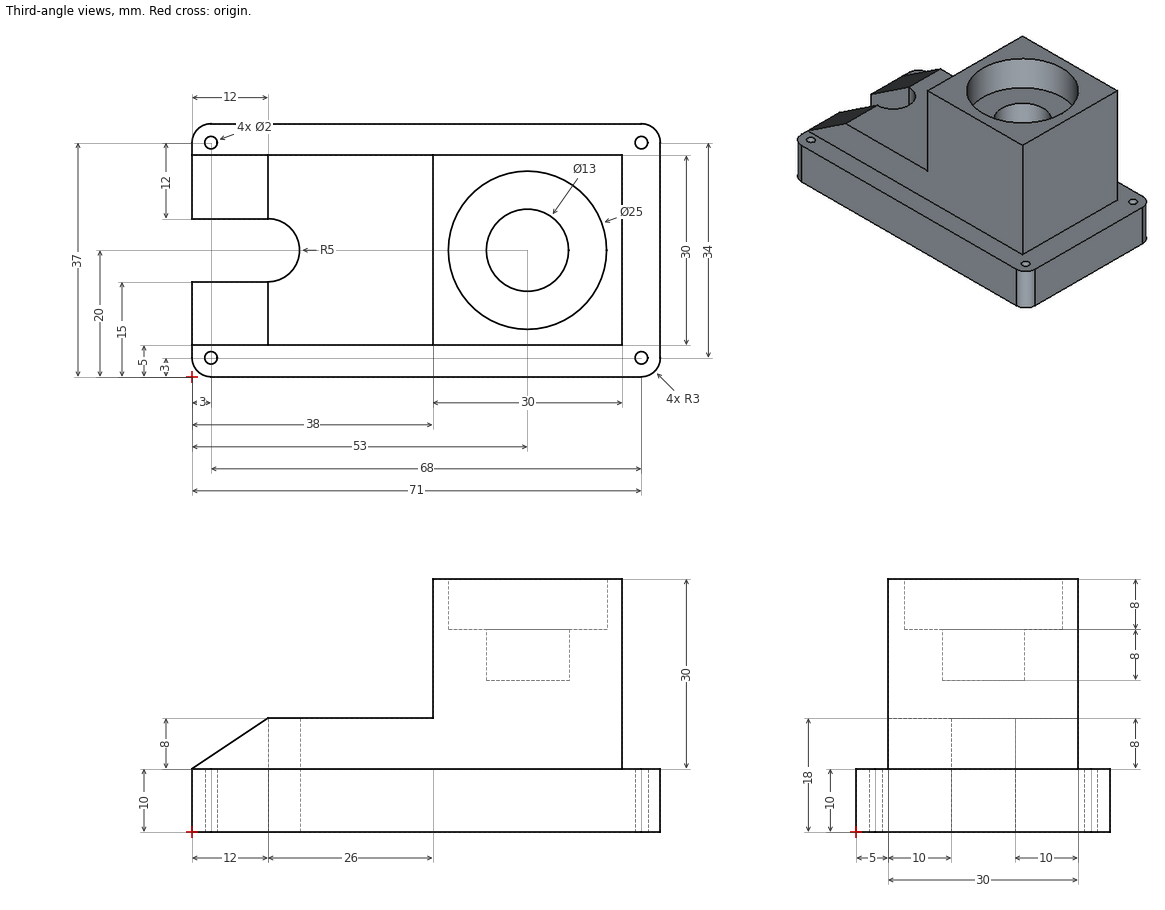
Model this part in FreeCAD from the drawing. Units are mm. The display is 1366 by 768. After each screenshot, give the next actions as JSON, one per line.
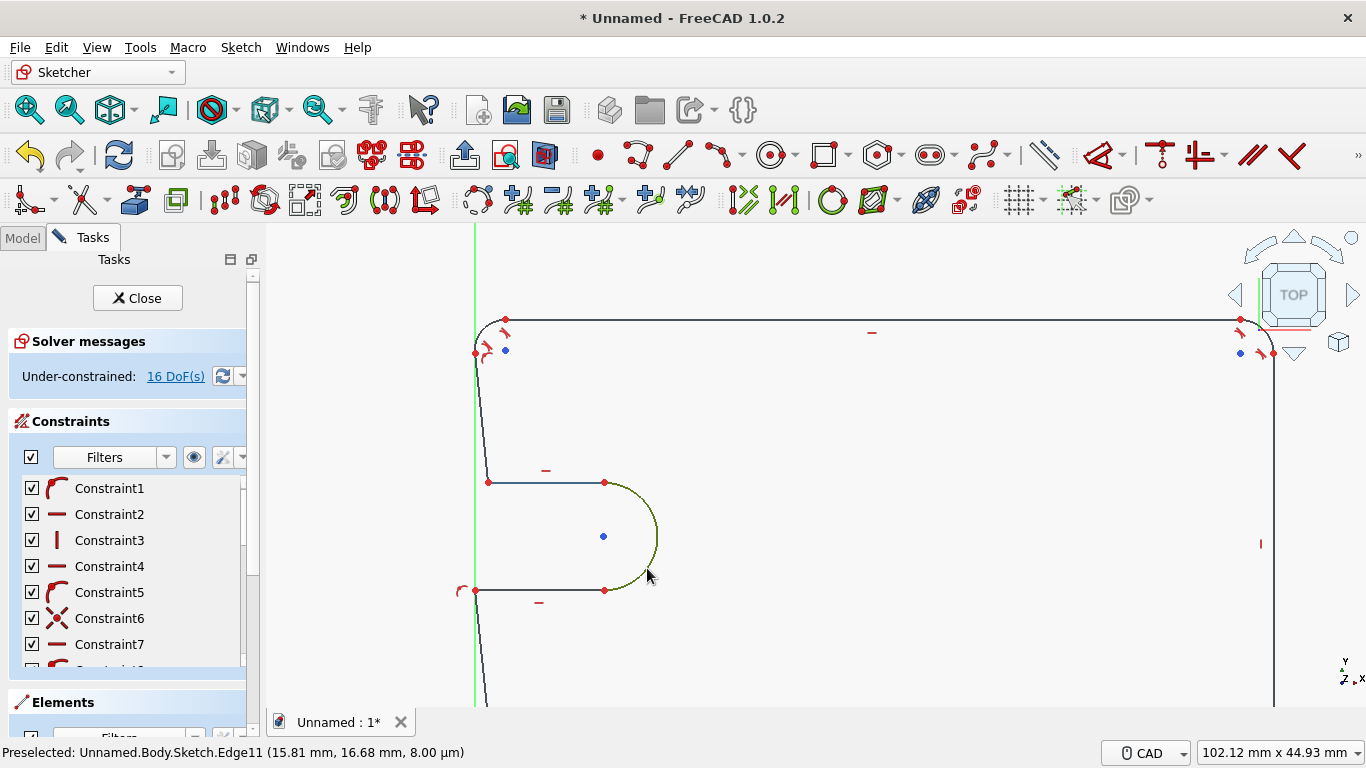
{"action": "key", "text": "t"}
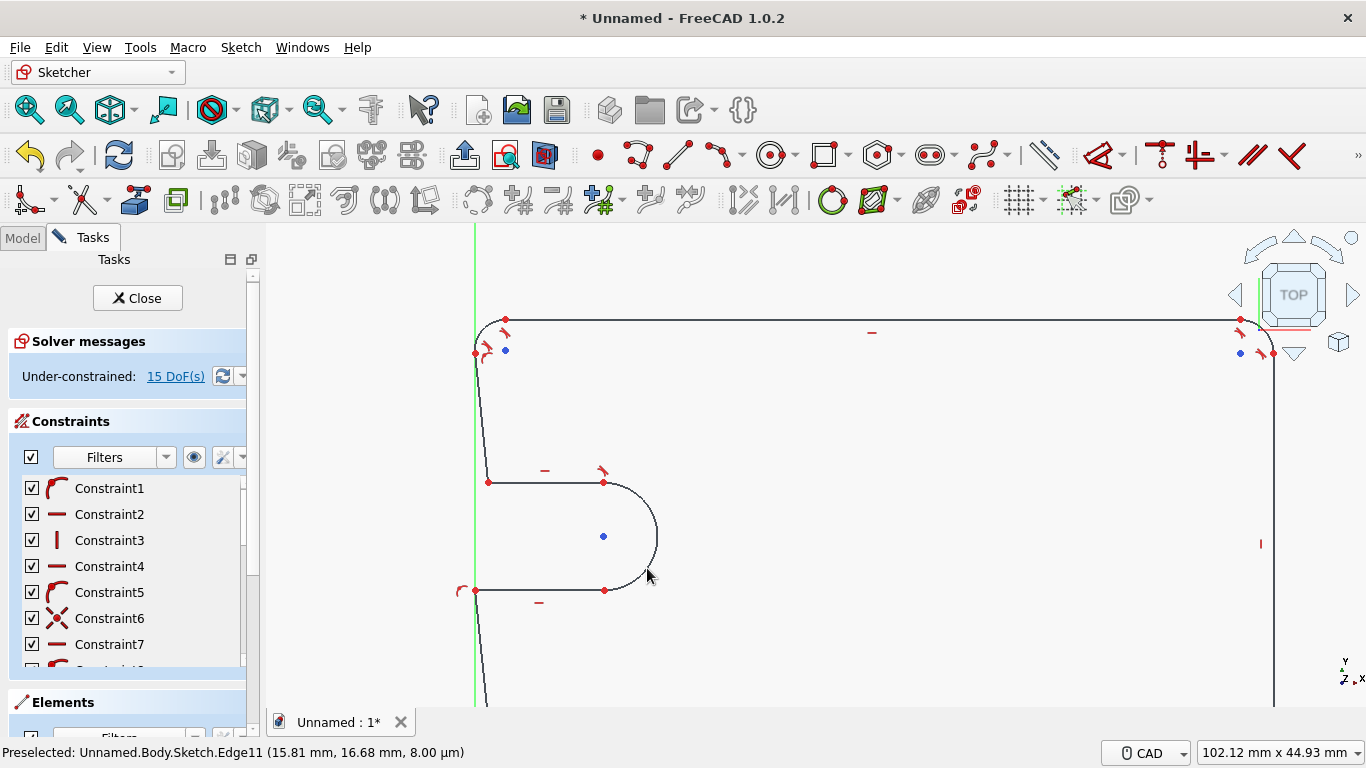
{"action": "left_click", "coordinate": [566, 590]}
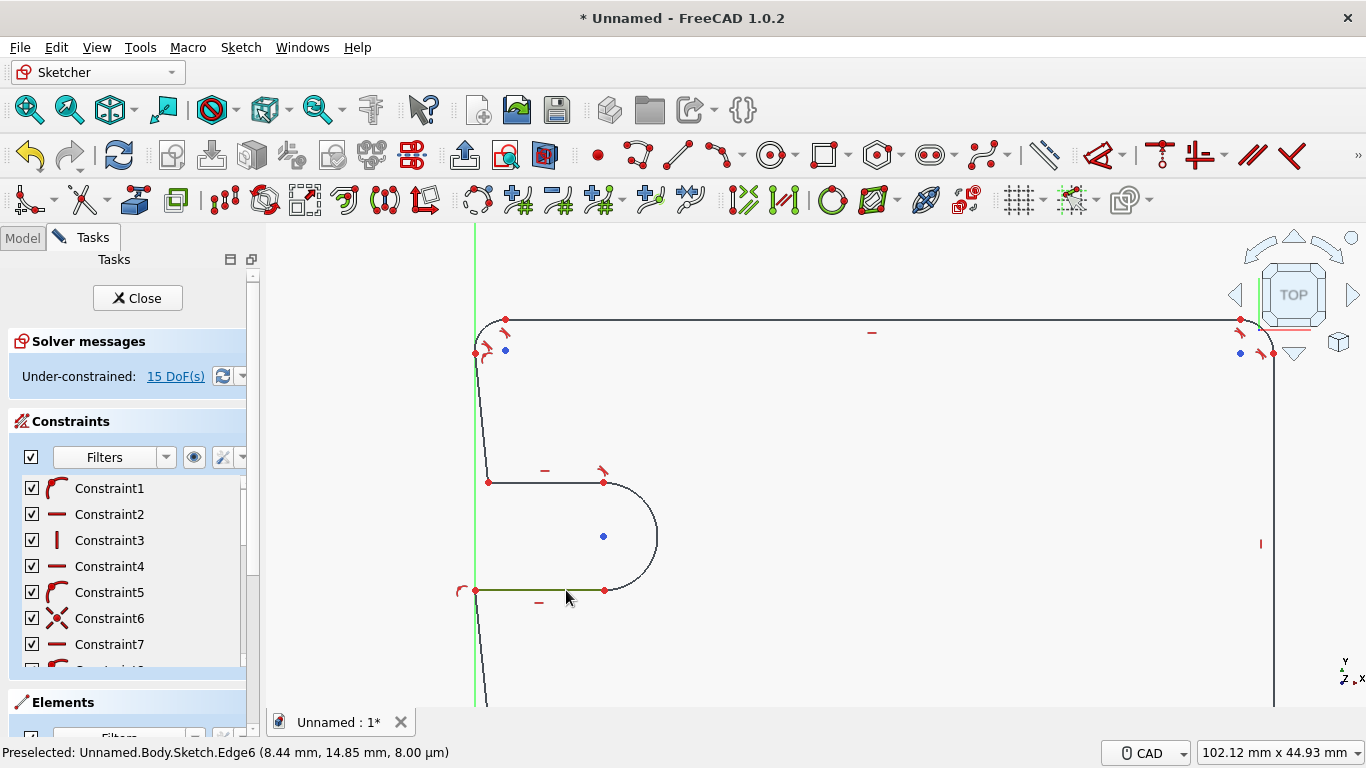
{"action": "left_click", "coordinate": [648, 568]}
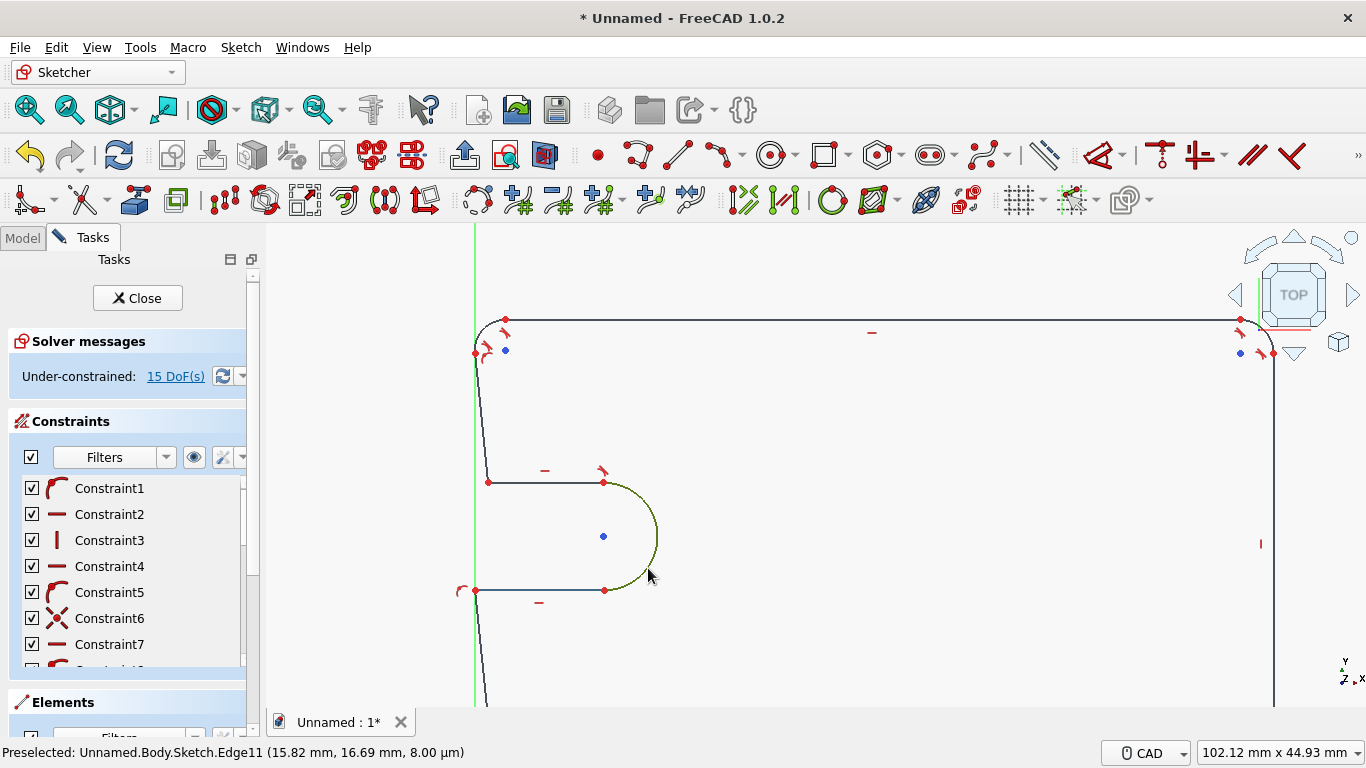
{"action": "key", "text": "t"}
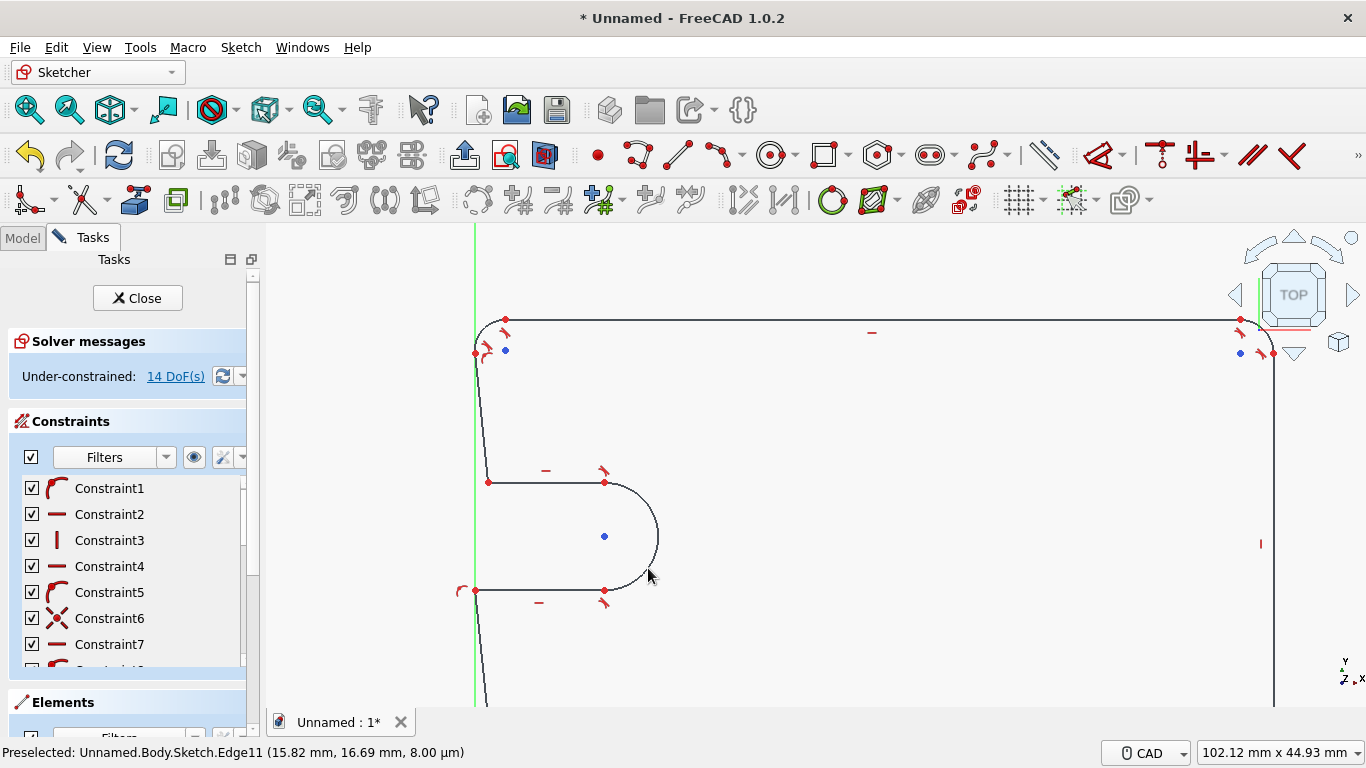
{"action": "left_click", "coordinate": [479, 629]}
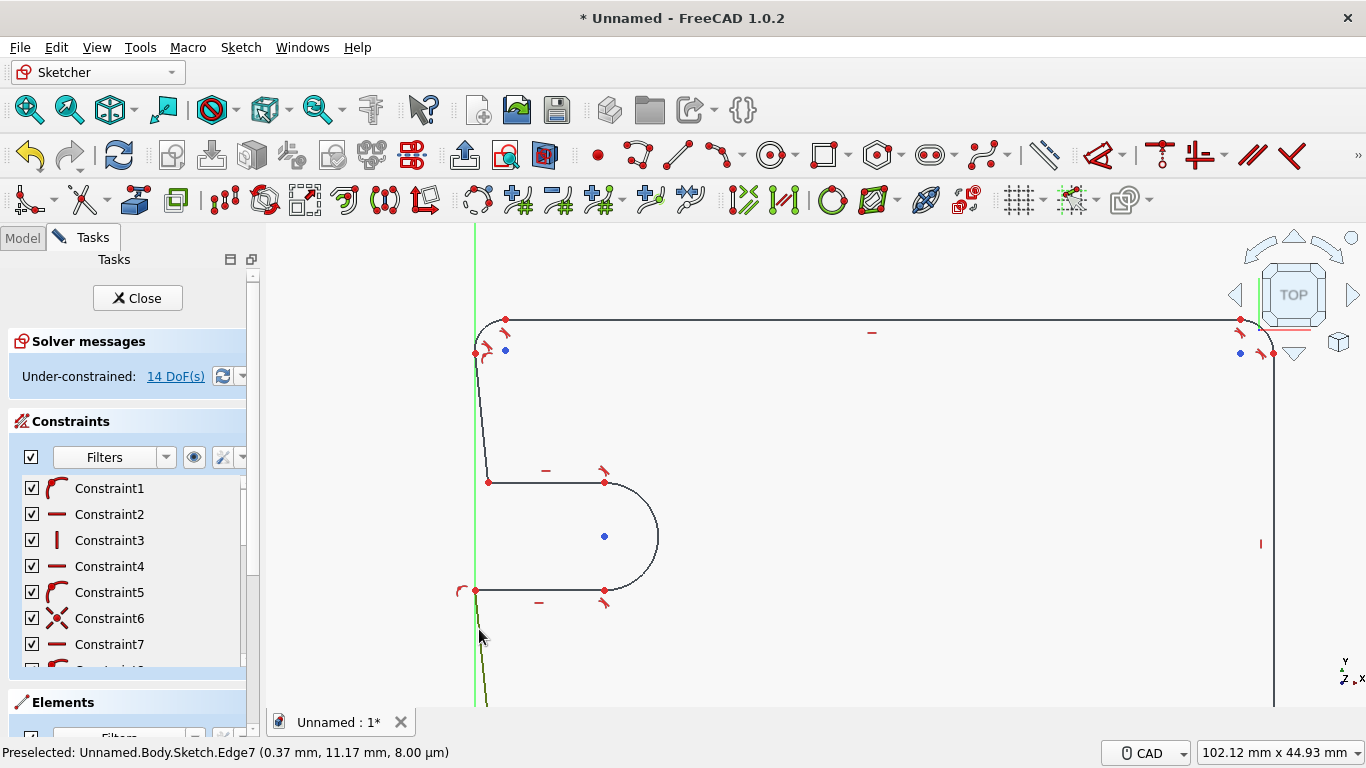
{"action": "scroll", "coordinate": [491, 323], "scroll_direction": "down", "scroll_amount": 2}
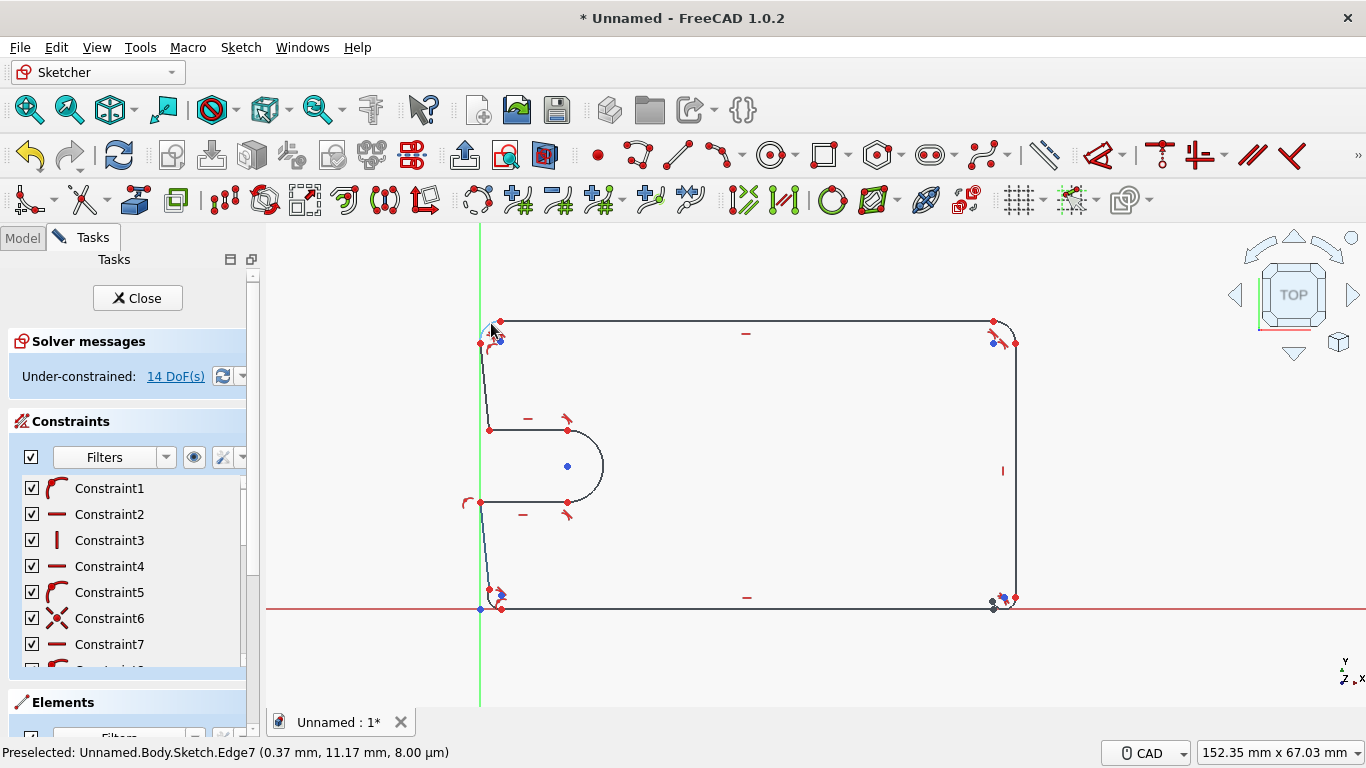
{"action": "scroll", "coordinate": [488, 598], "scroll_direction": "up", "scroll_amount": 4}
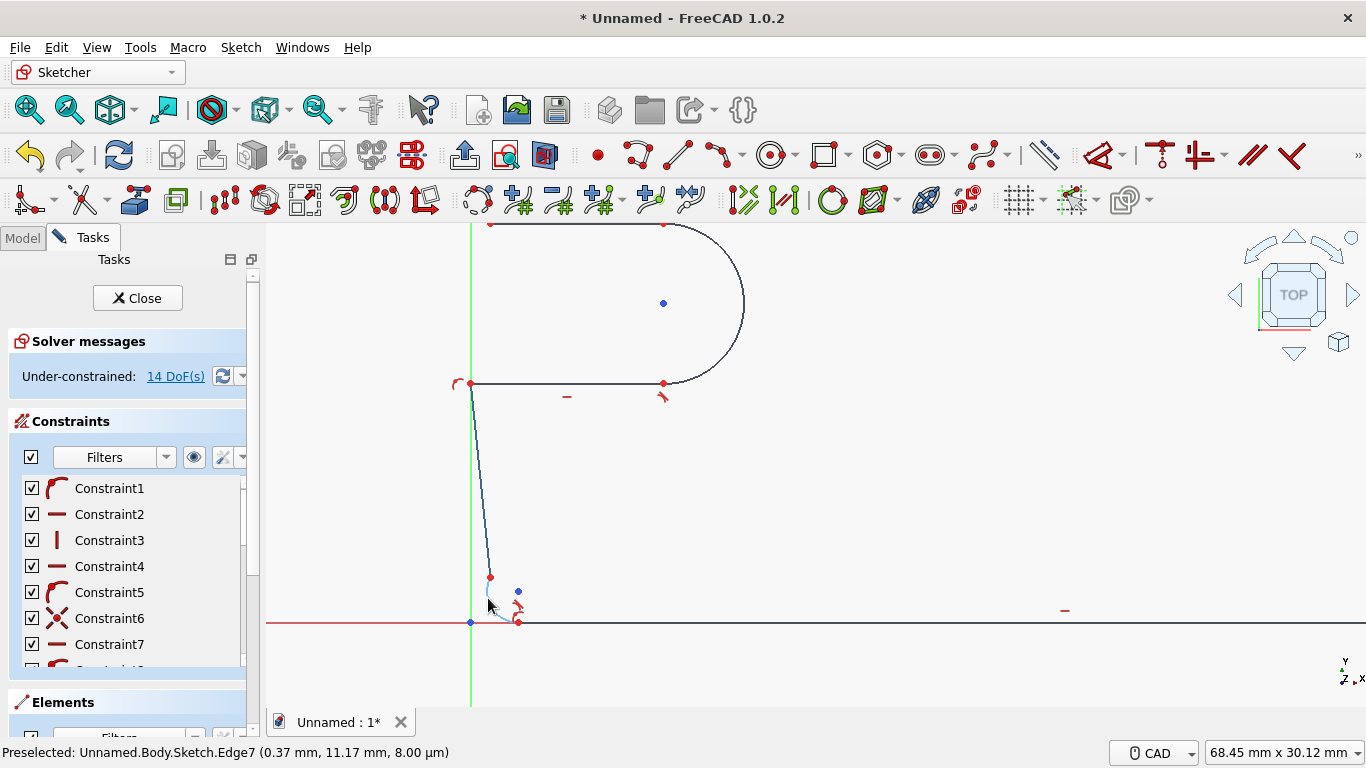
{"action": "left_click", "coordinate": [487, 596]}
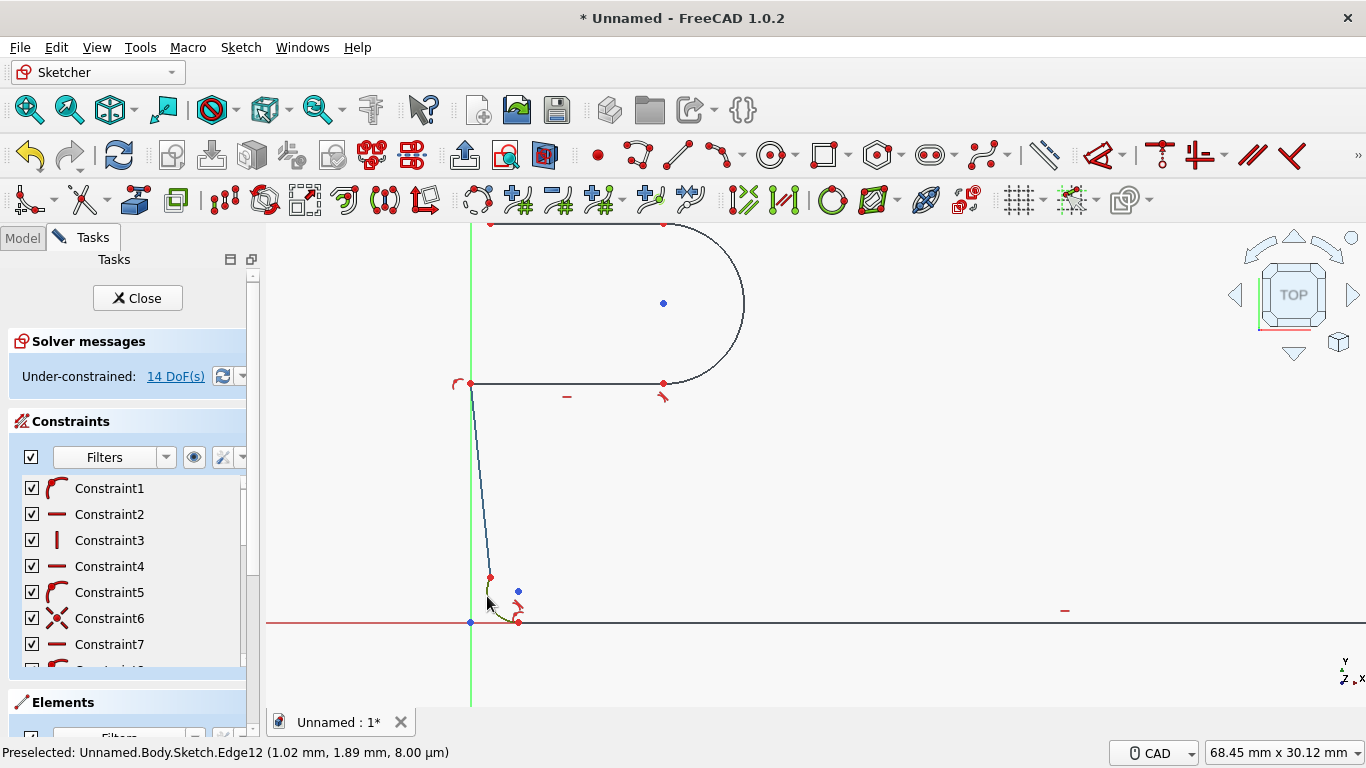
{"action": "key", "text": "t"}